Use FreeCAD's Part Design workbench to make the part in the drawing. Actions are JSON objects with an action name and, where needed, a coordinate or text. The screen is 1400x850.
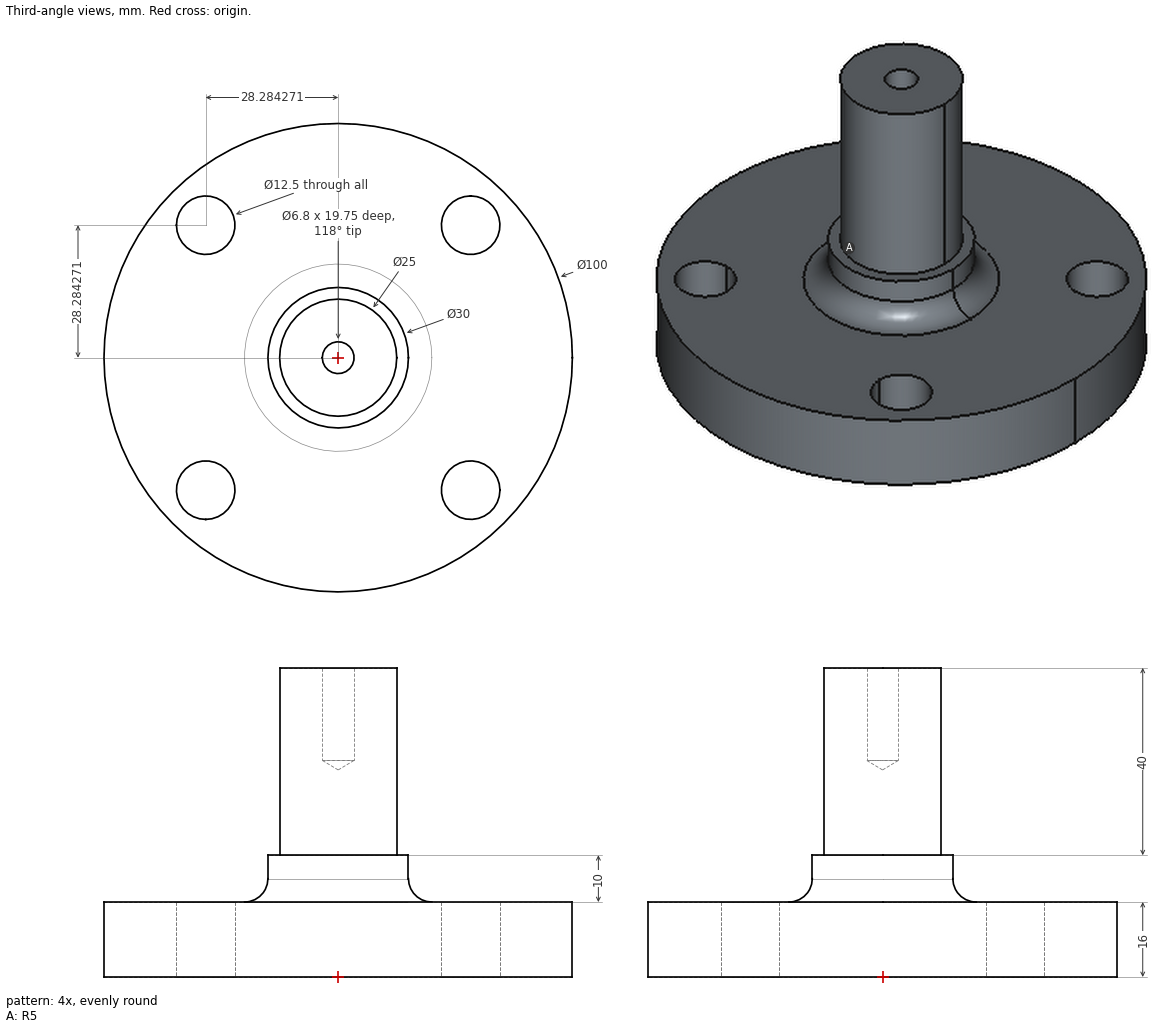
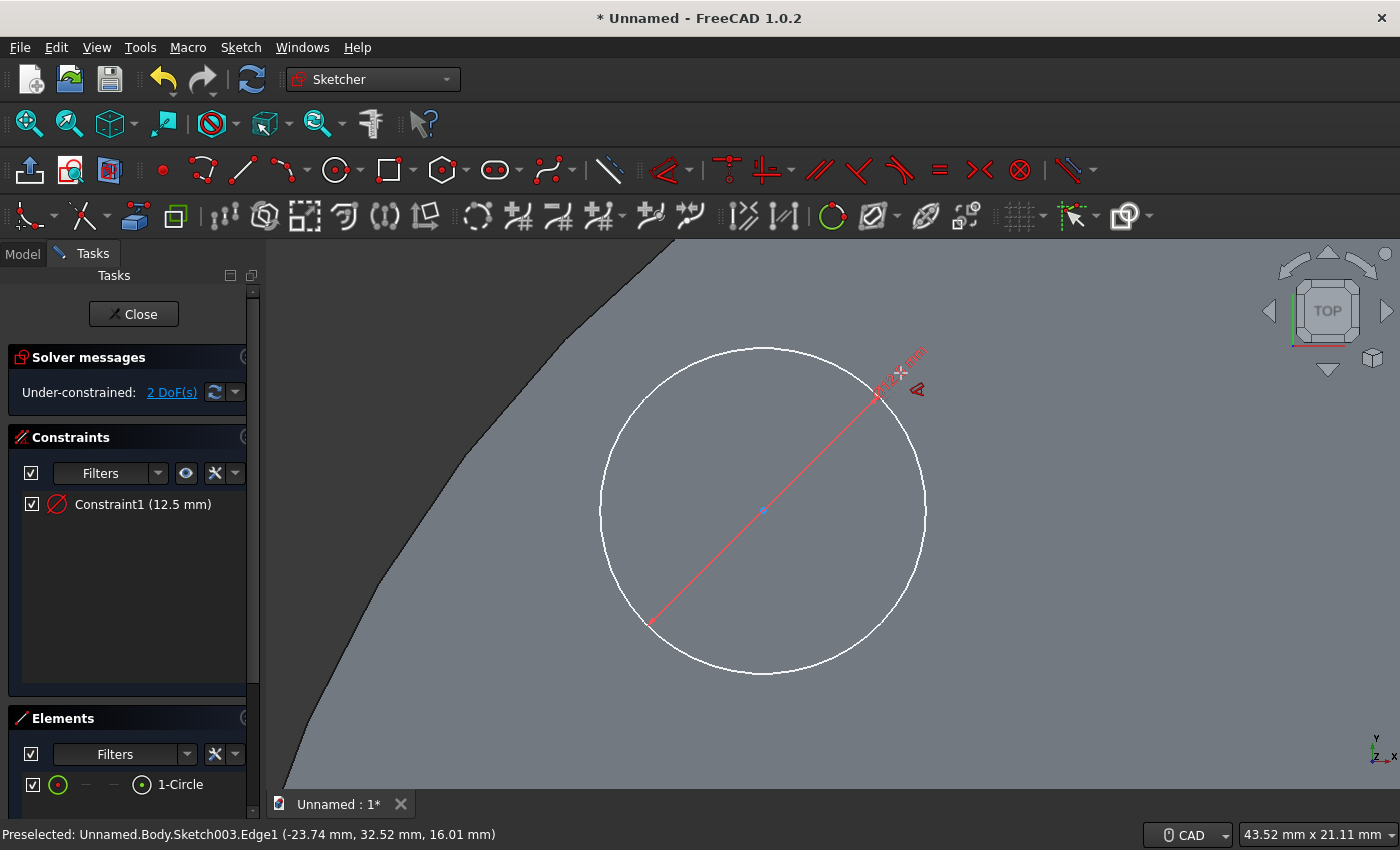
{"action": "left_click", "coordinate": [763, 511]}
{"action": "left_click", "coordinate": [999, 477]}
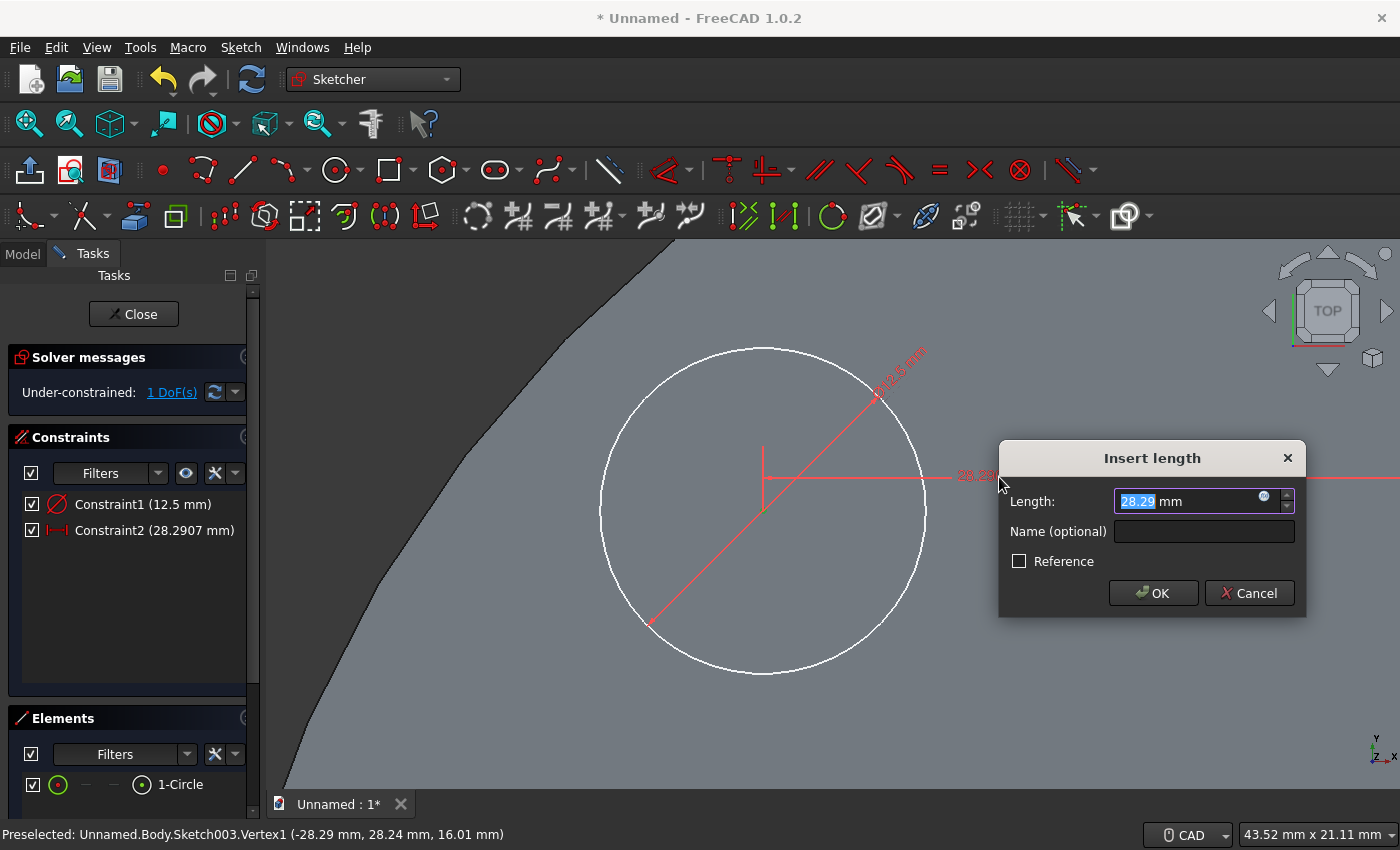
{"action": "type", "text": "28.284271"}
{"action": "key", "text": "Return"}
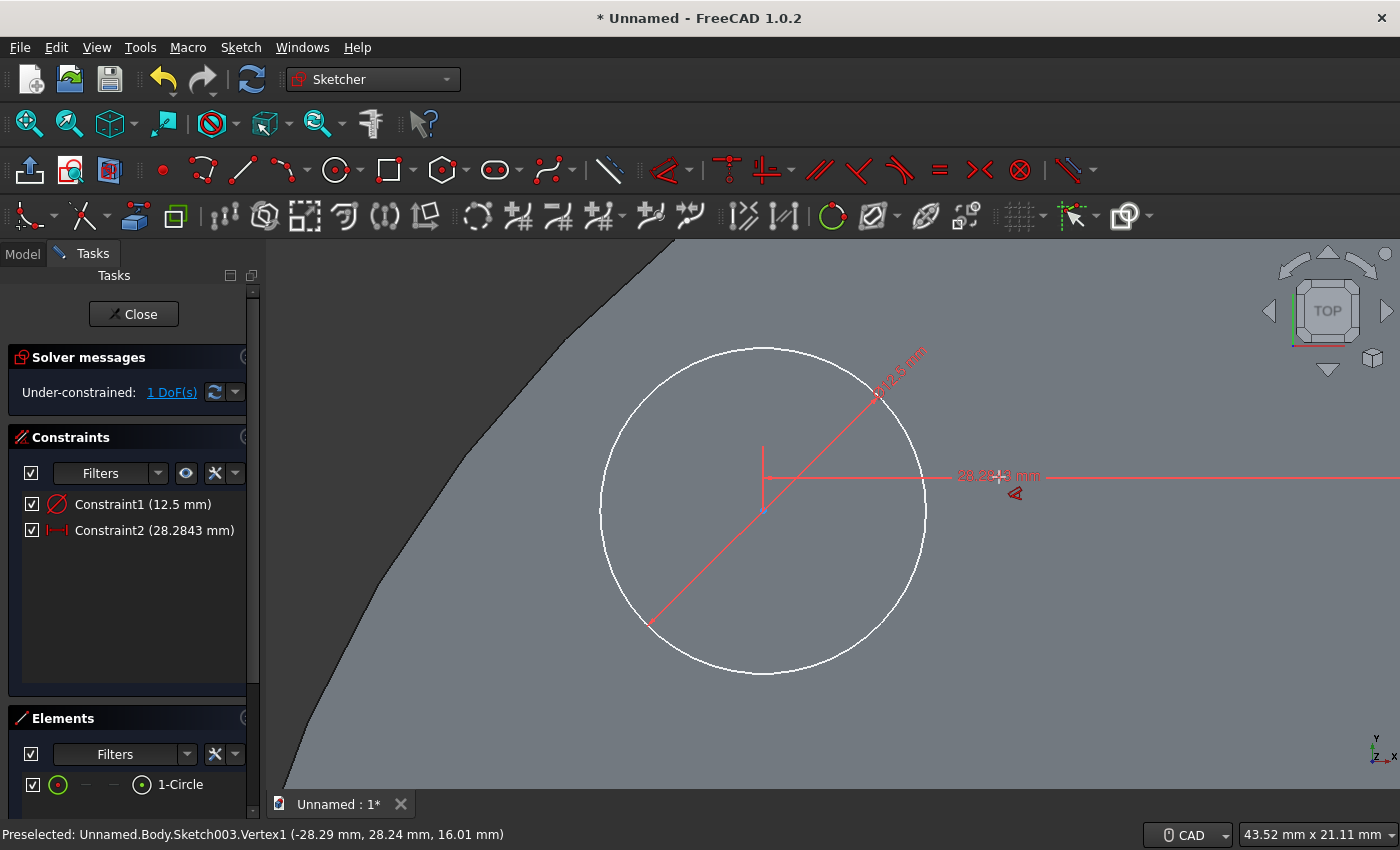
{"action": "left_click", "coordinate": [763, 511]}
{"action": "left_click", "coordinate": [729, 636]}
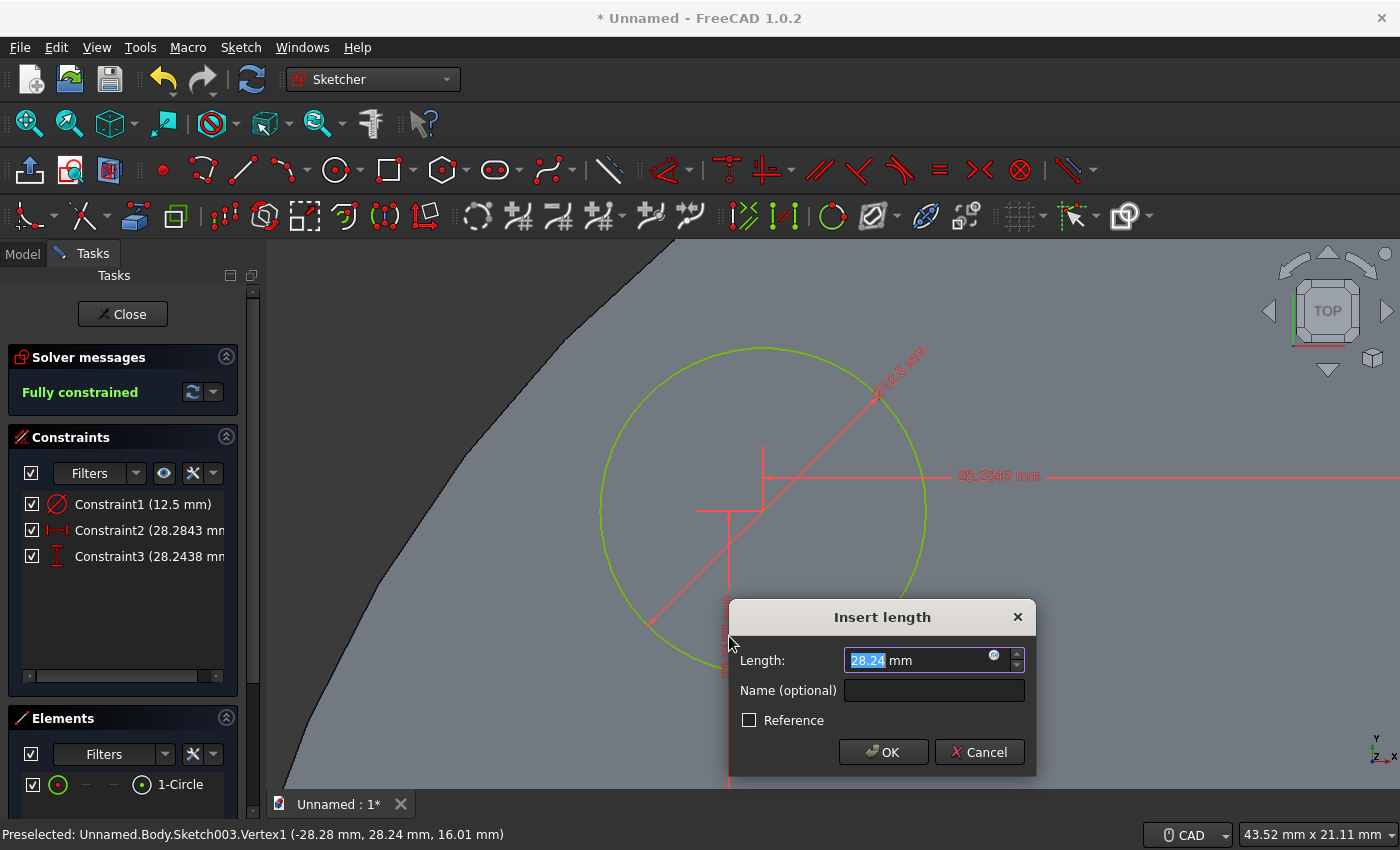
{"action": "type", "text": "28.284271"}
{"action": "key", "text": "Return"}
{"action": "key", "text": "Escape"}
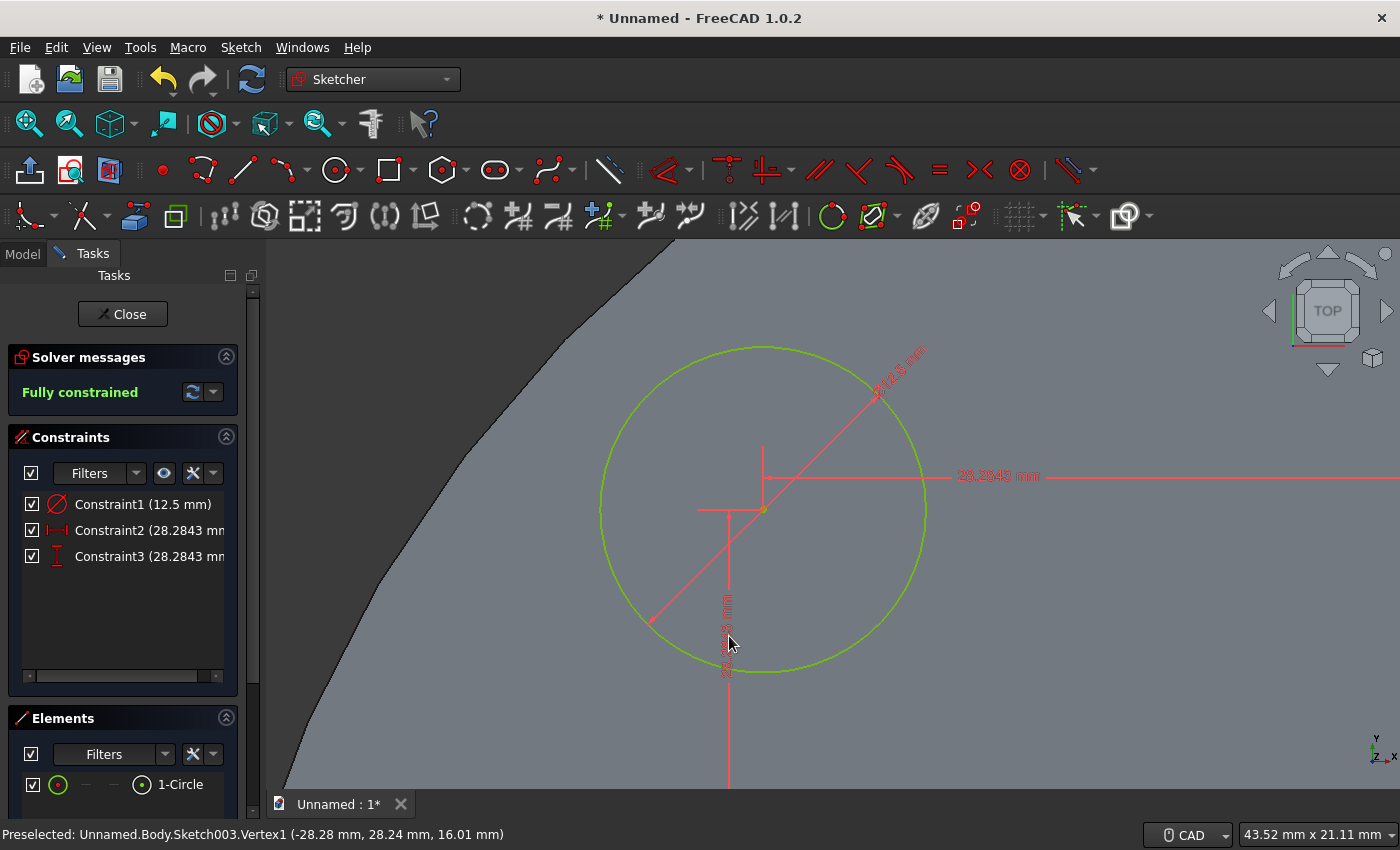
{"action": "left_click", "coordinate": [123, 314]}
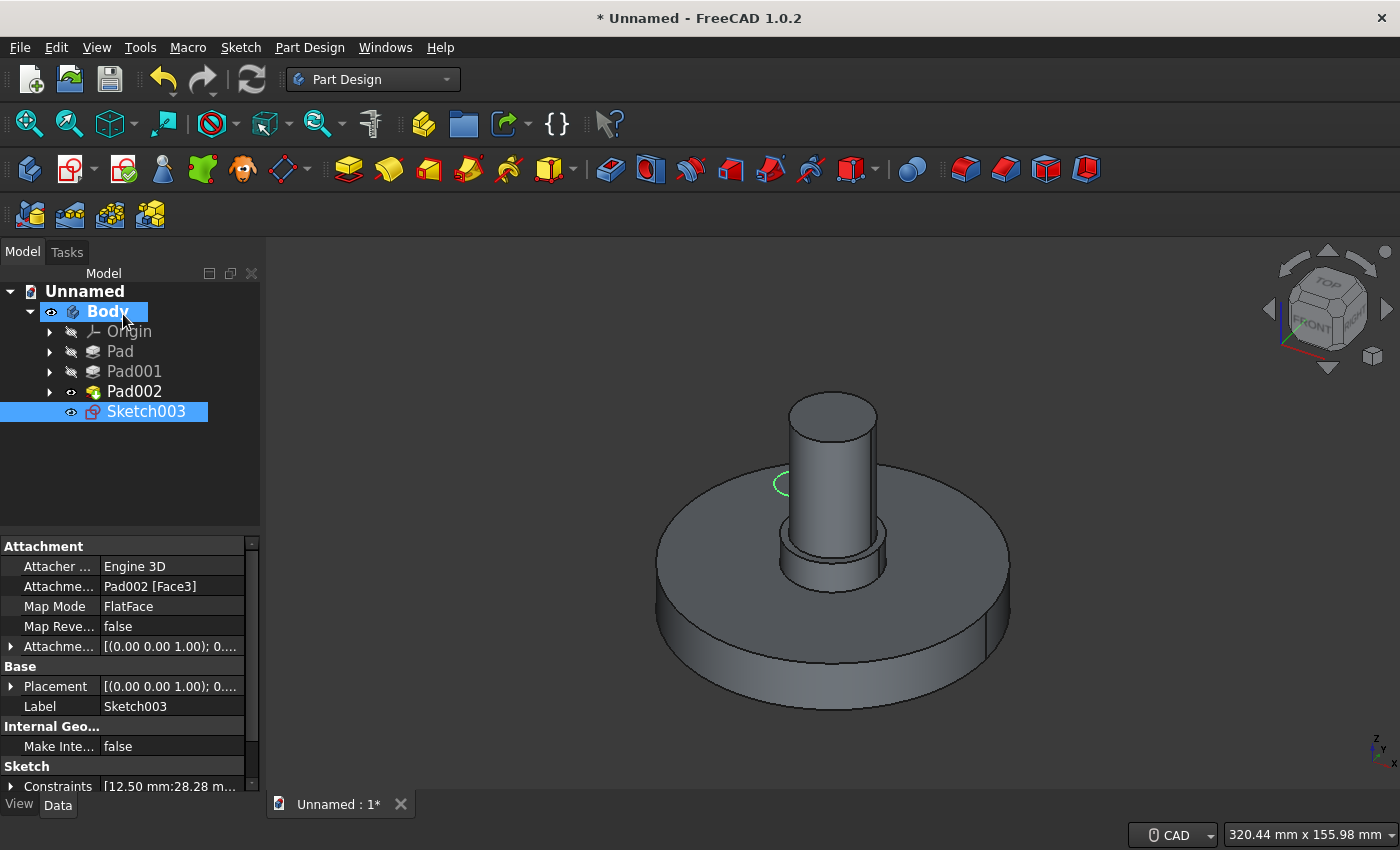
{"action": "left_click", "coordinate": [652, 170]}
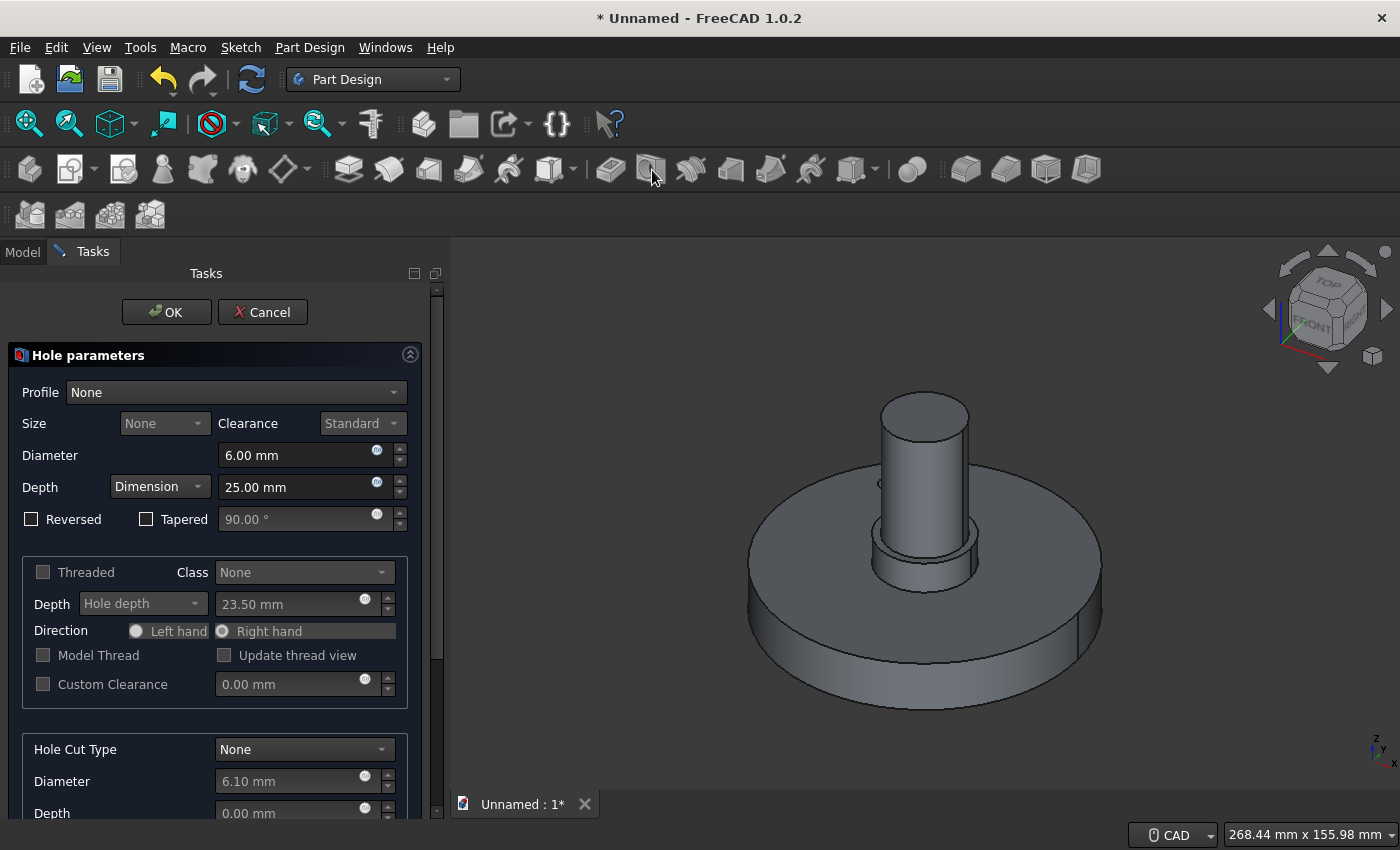
{"action": "triple_click", "coordinate": [305, 455]}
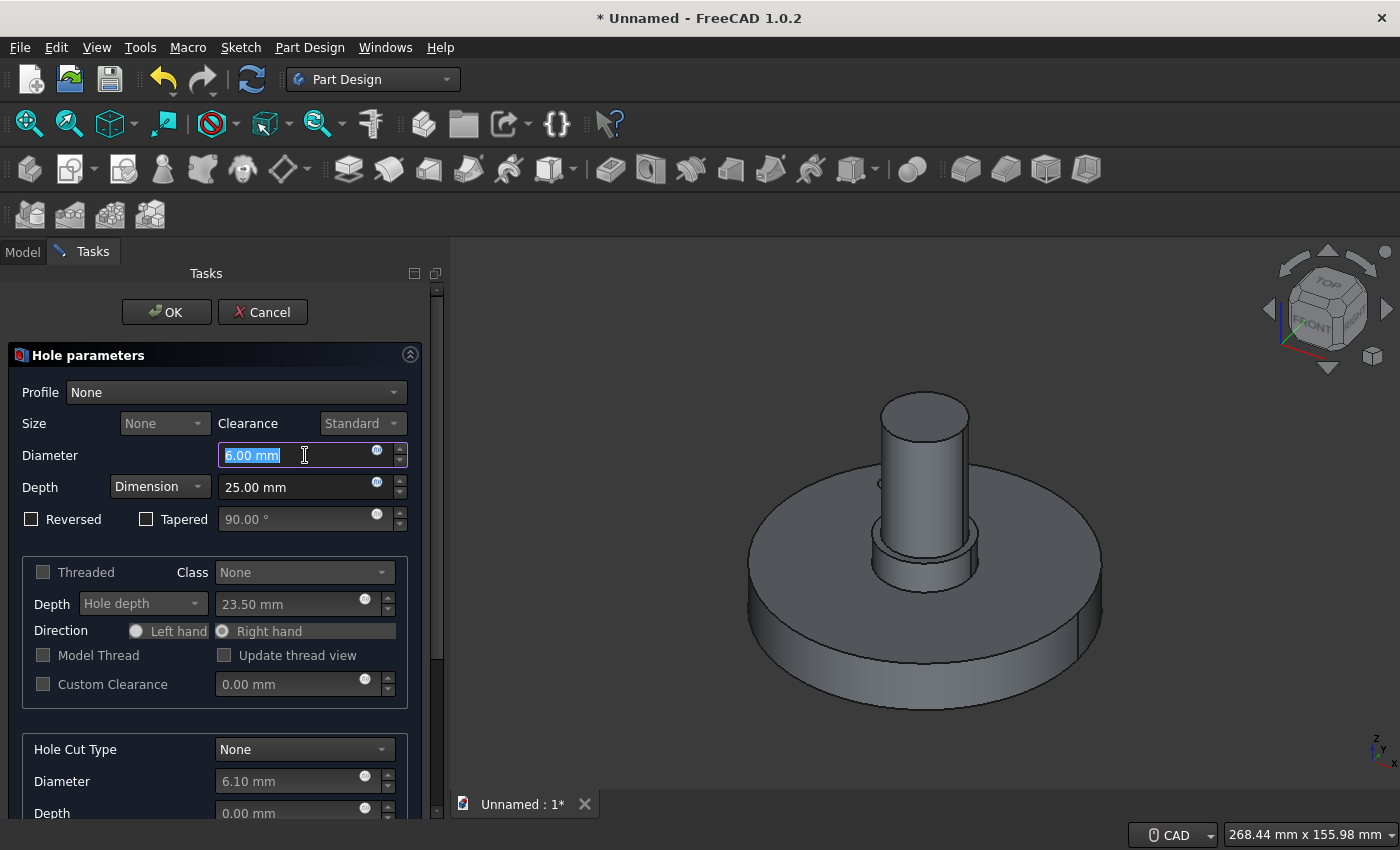
{"action": "type", "text": "12.5"}
{"action": "key", "text": "Tab"}